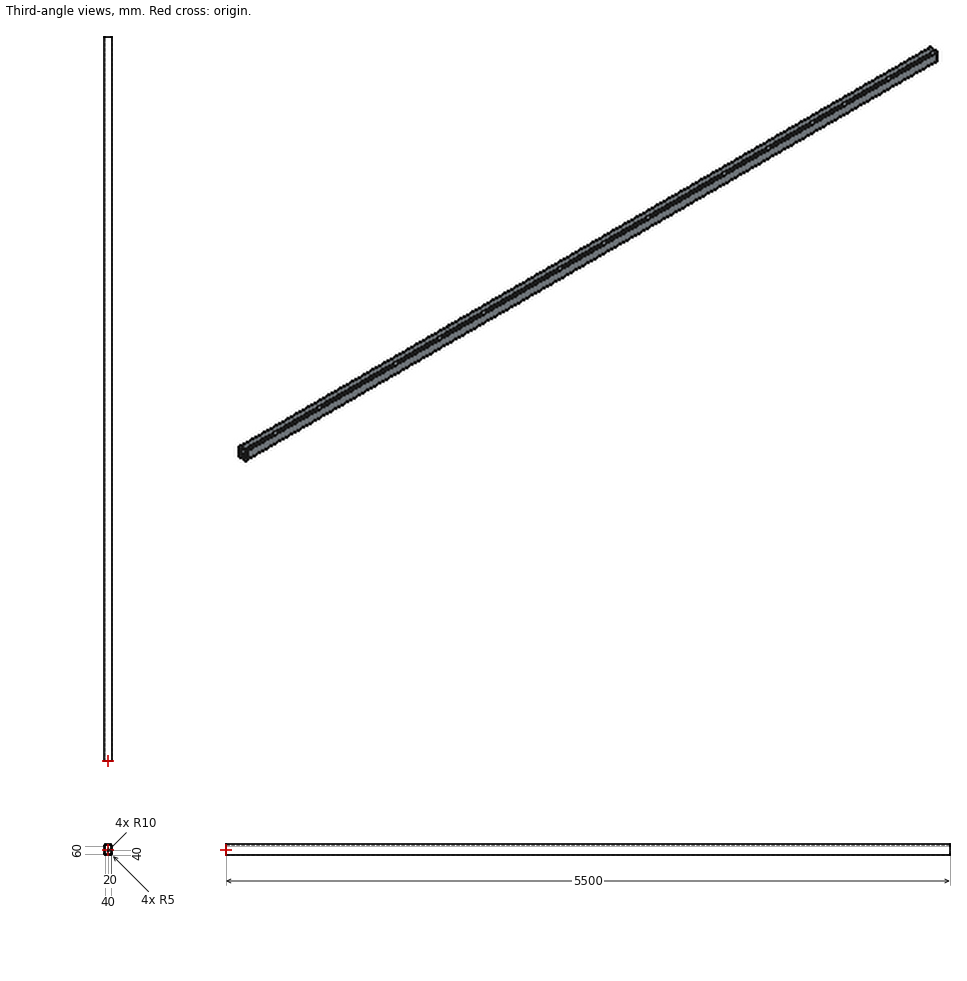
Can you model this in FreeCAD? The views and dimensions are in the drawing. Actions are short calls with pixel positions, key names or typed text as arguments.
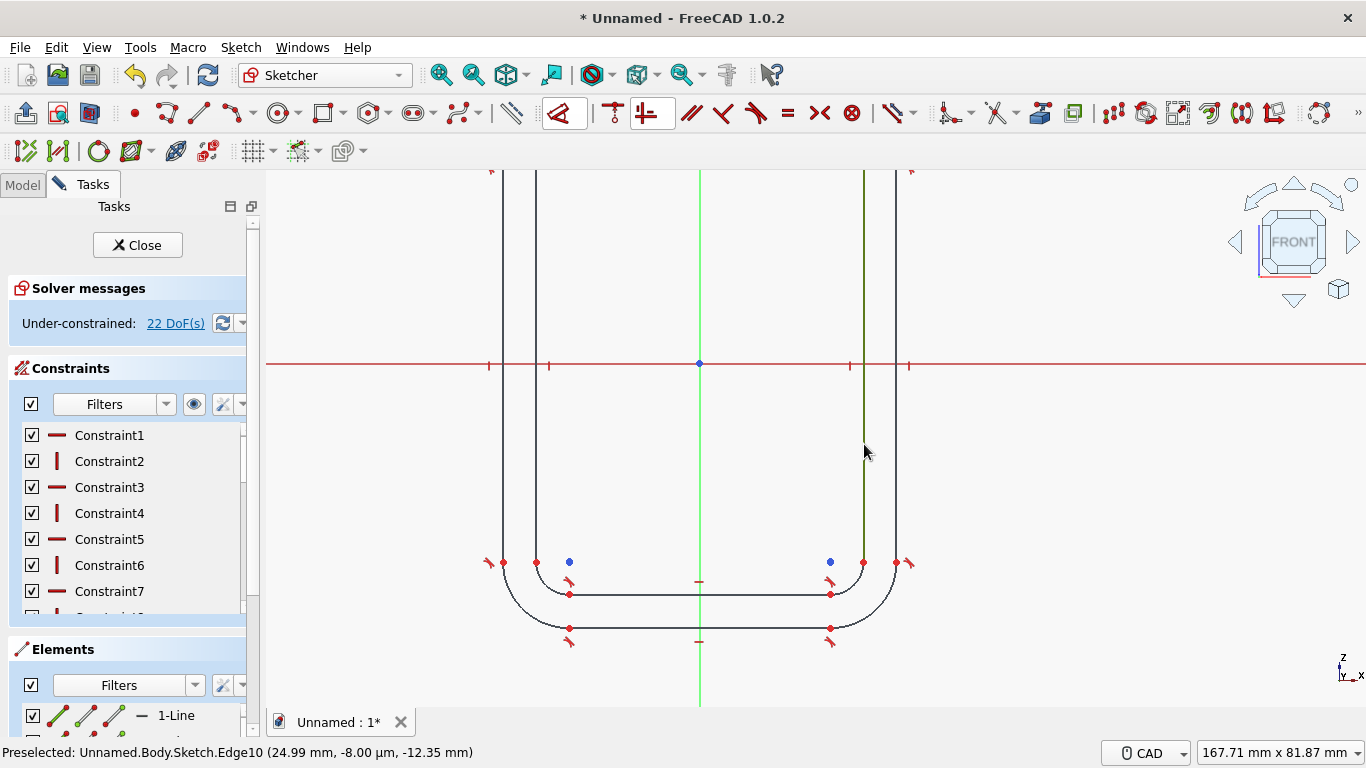
click(845, 591)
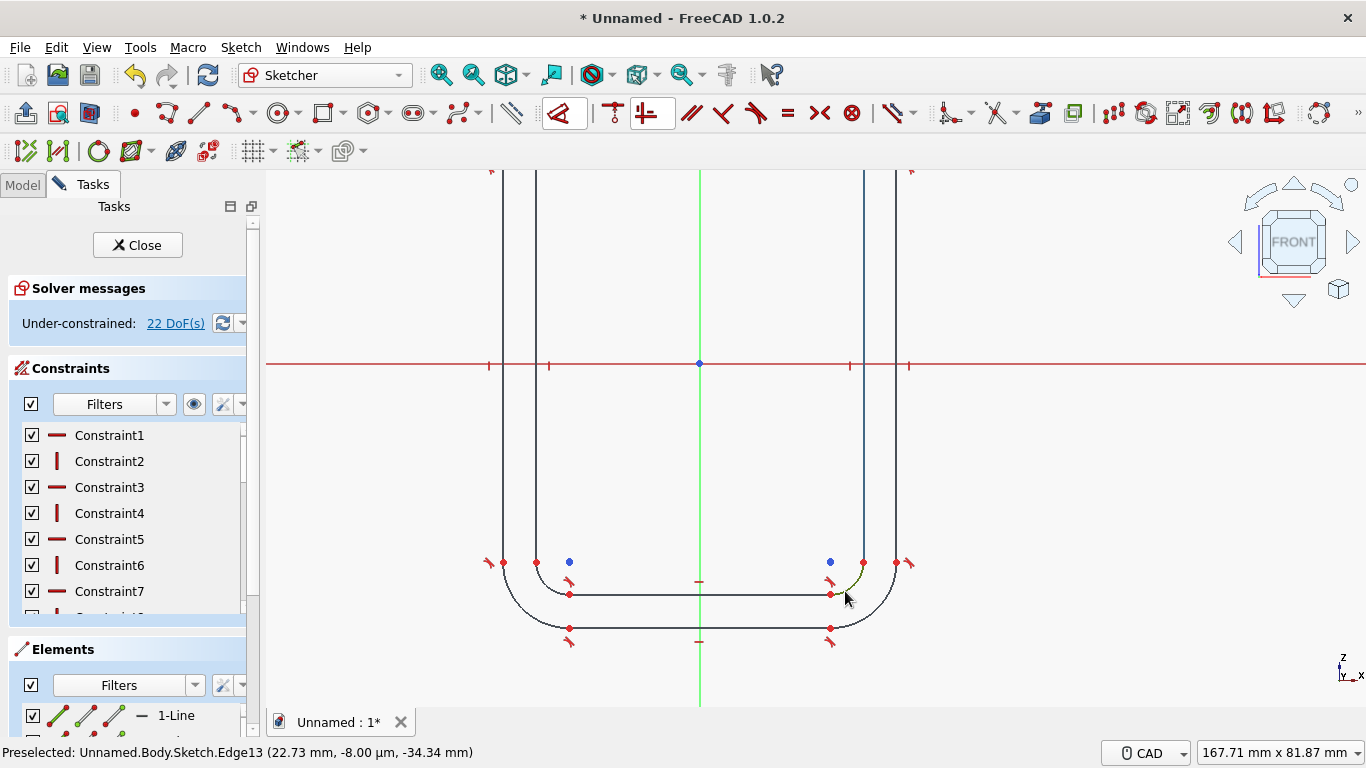
click(756, 114)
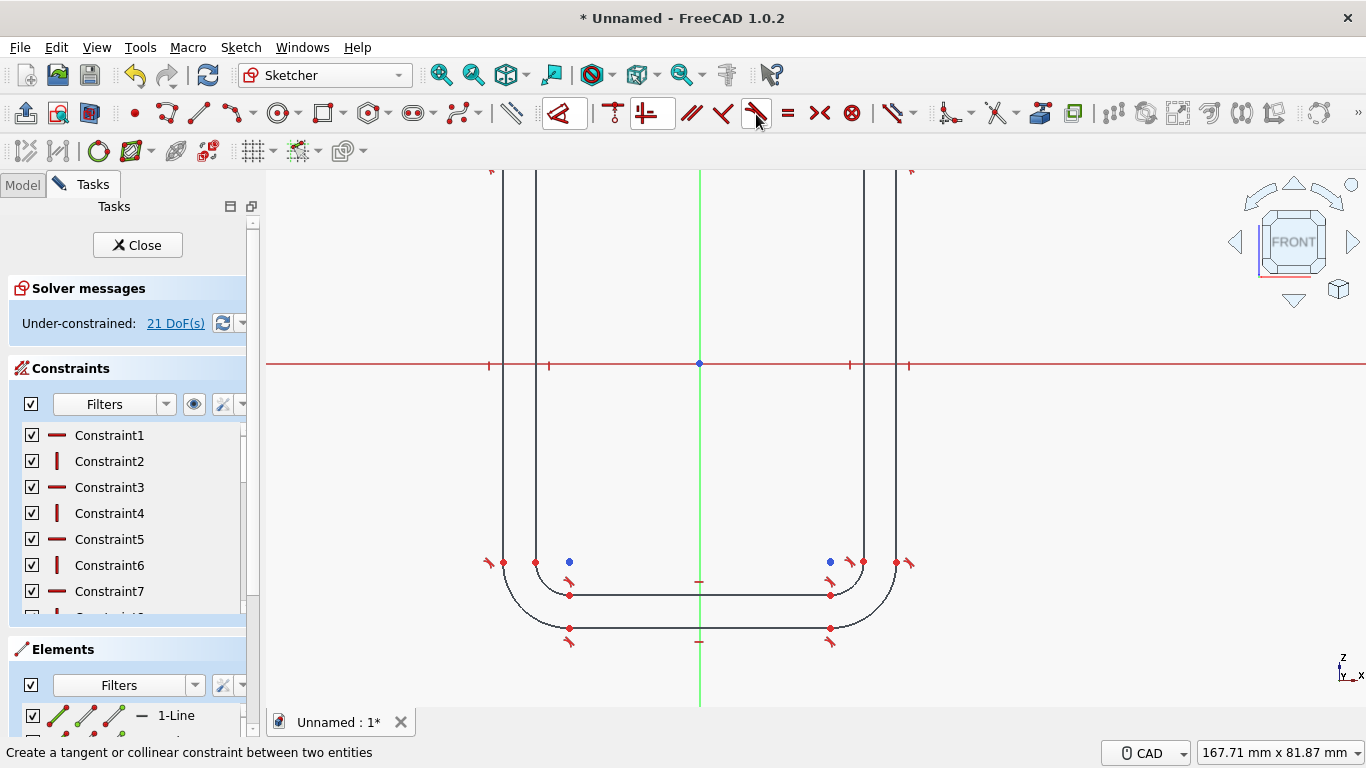
click(864, 444)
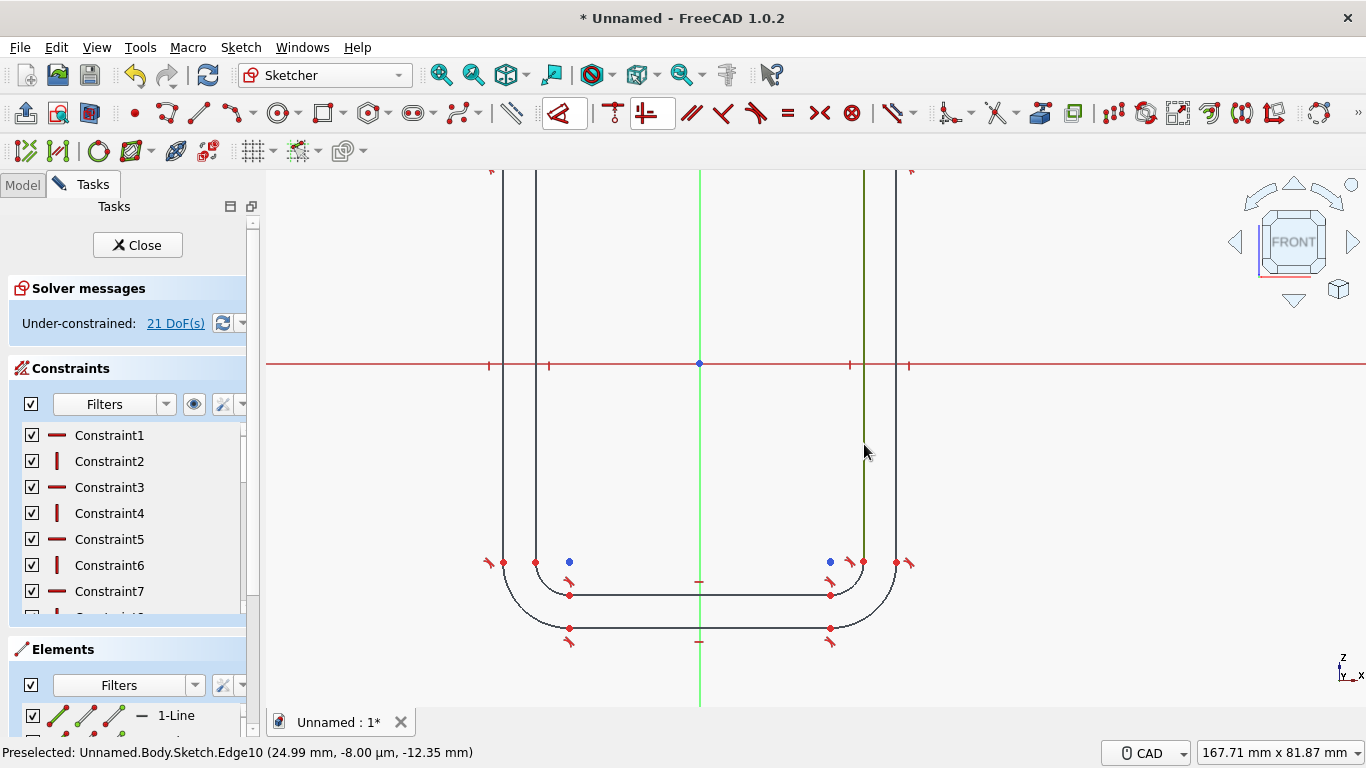
scroll(844, 590, down, 2)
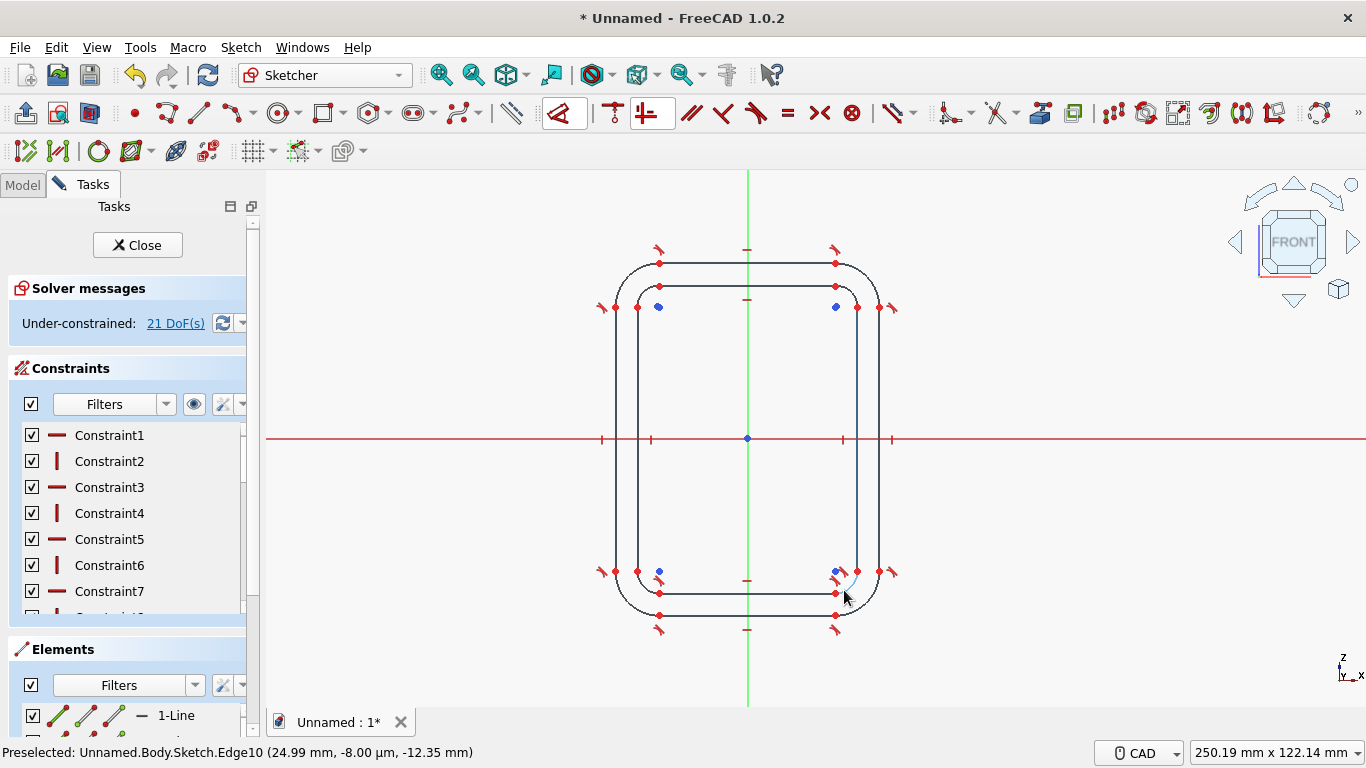
scroll(855, 297, up, 2)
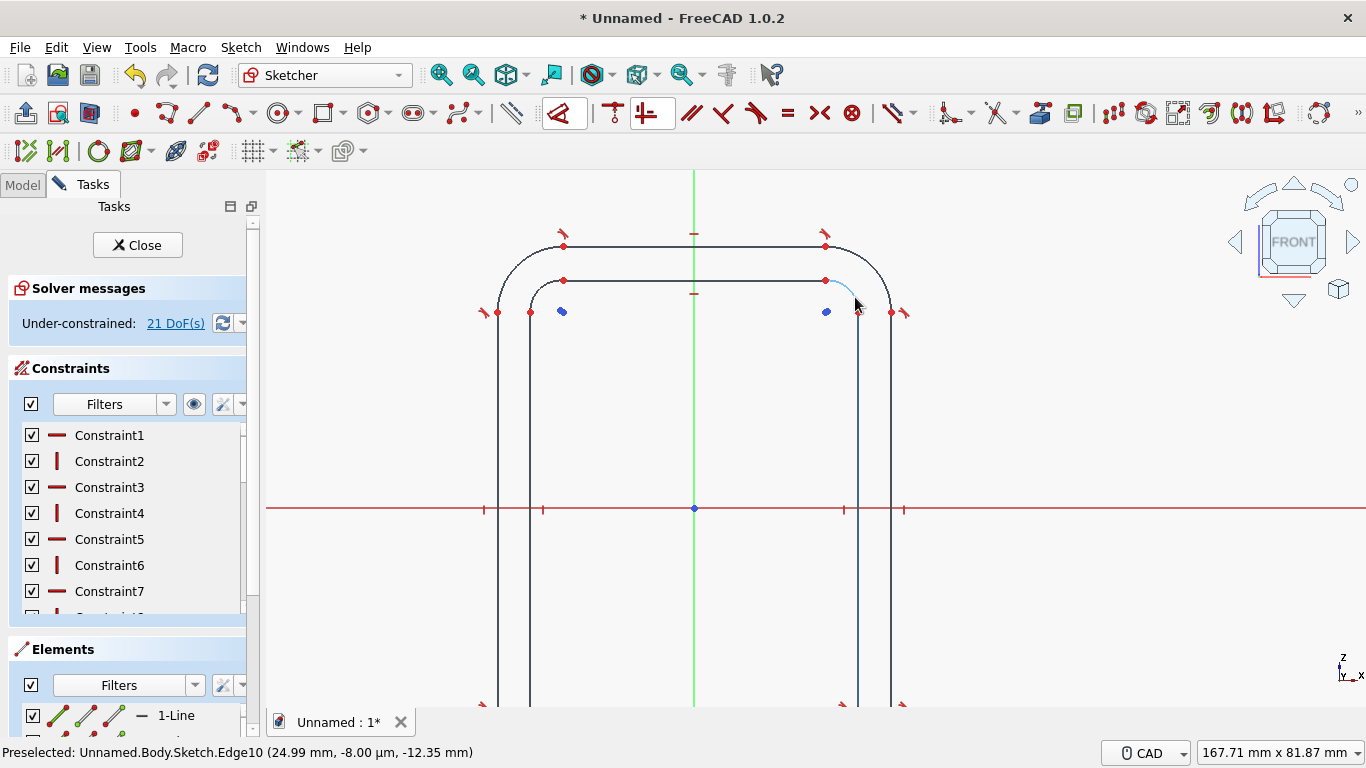
click(855, 297)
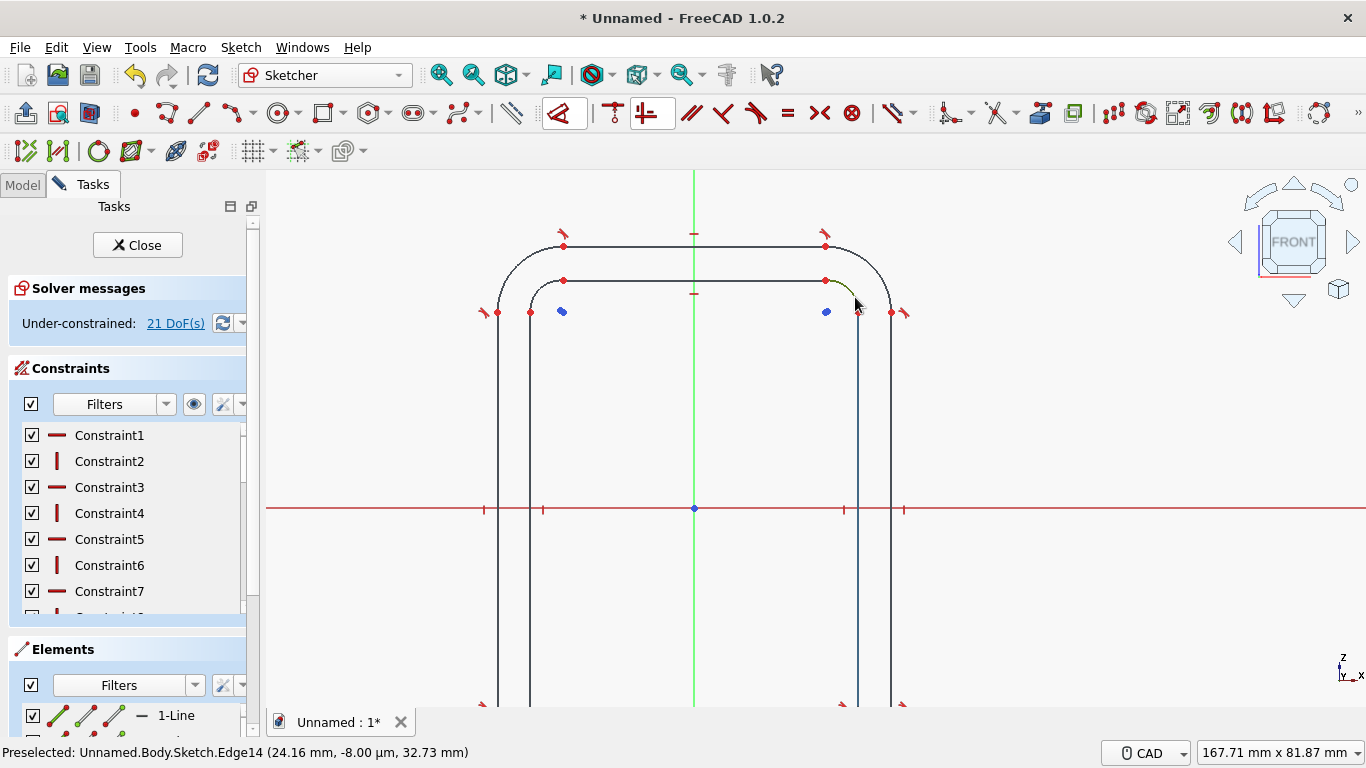
click(756, 114)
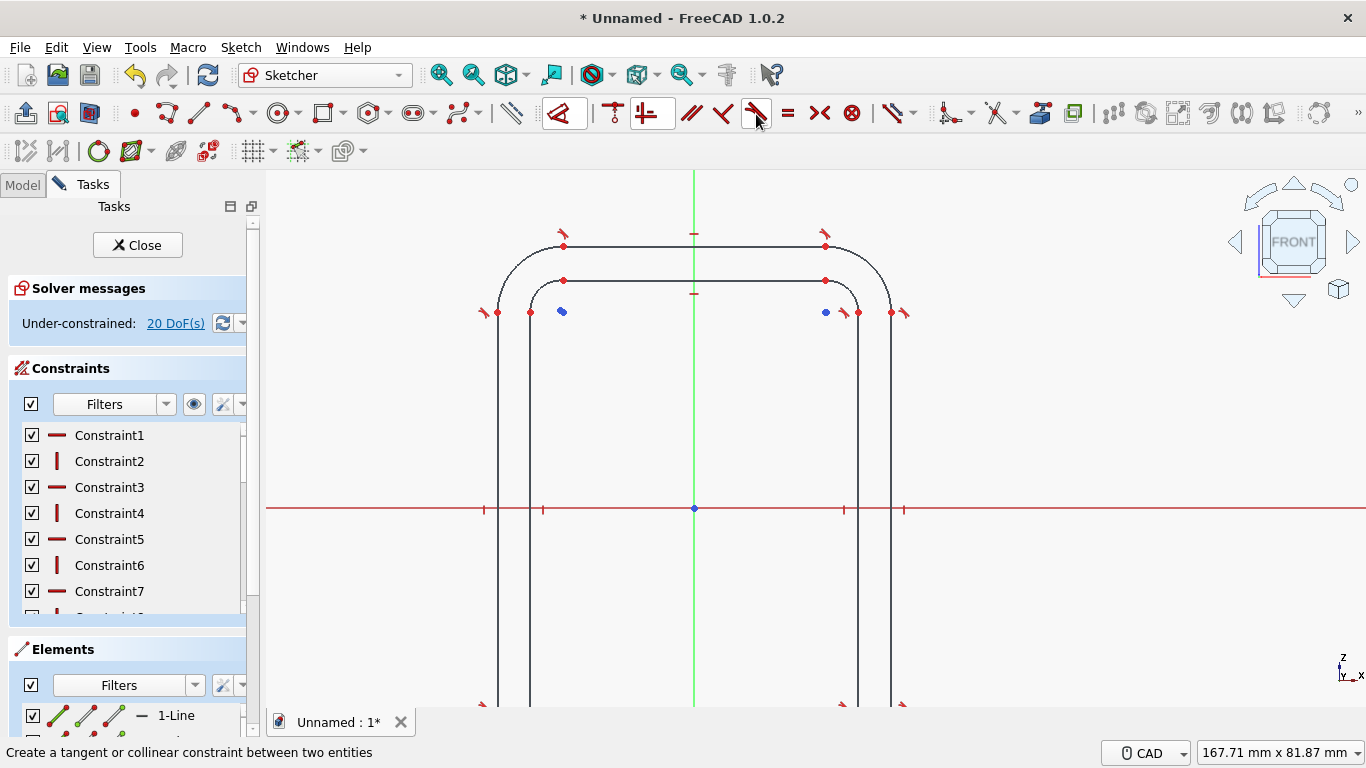
click(747, 281)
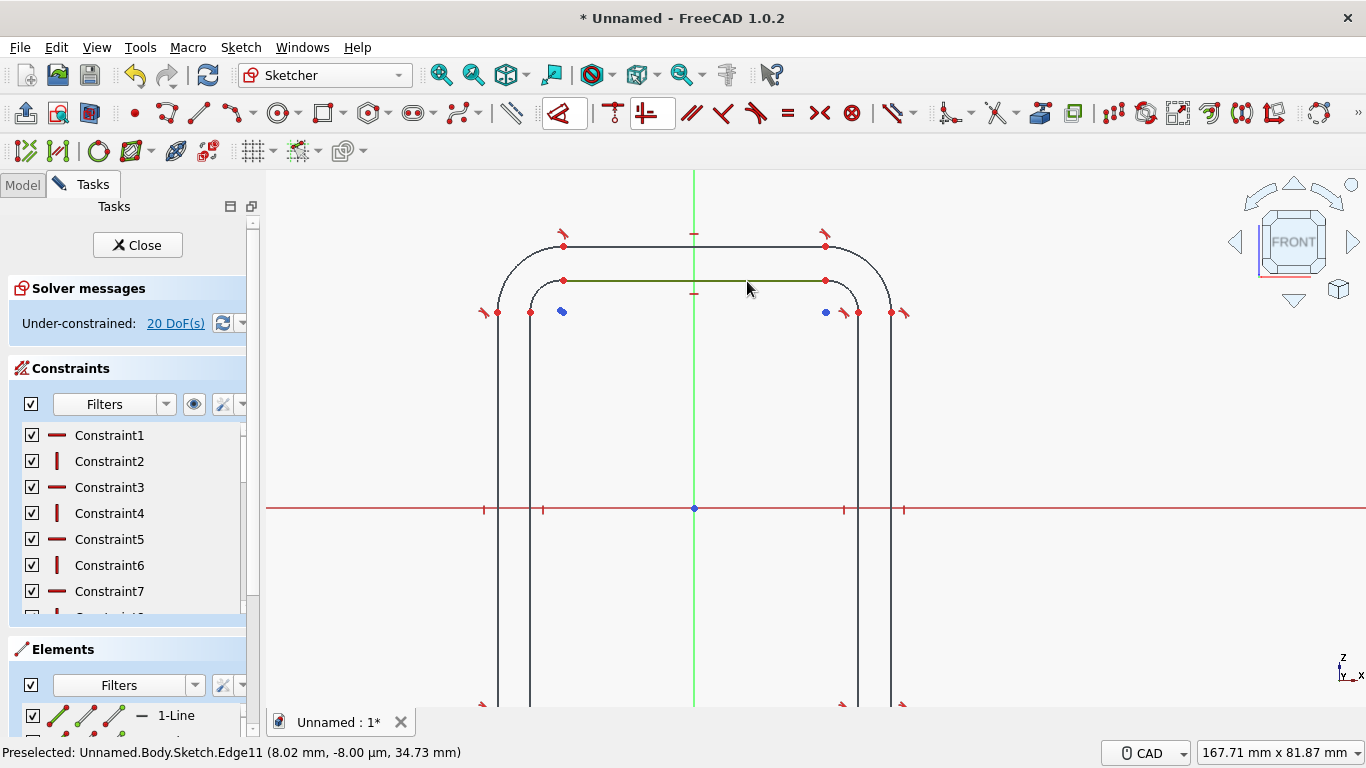
click(855, 297)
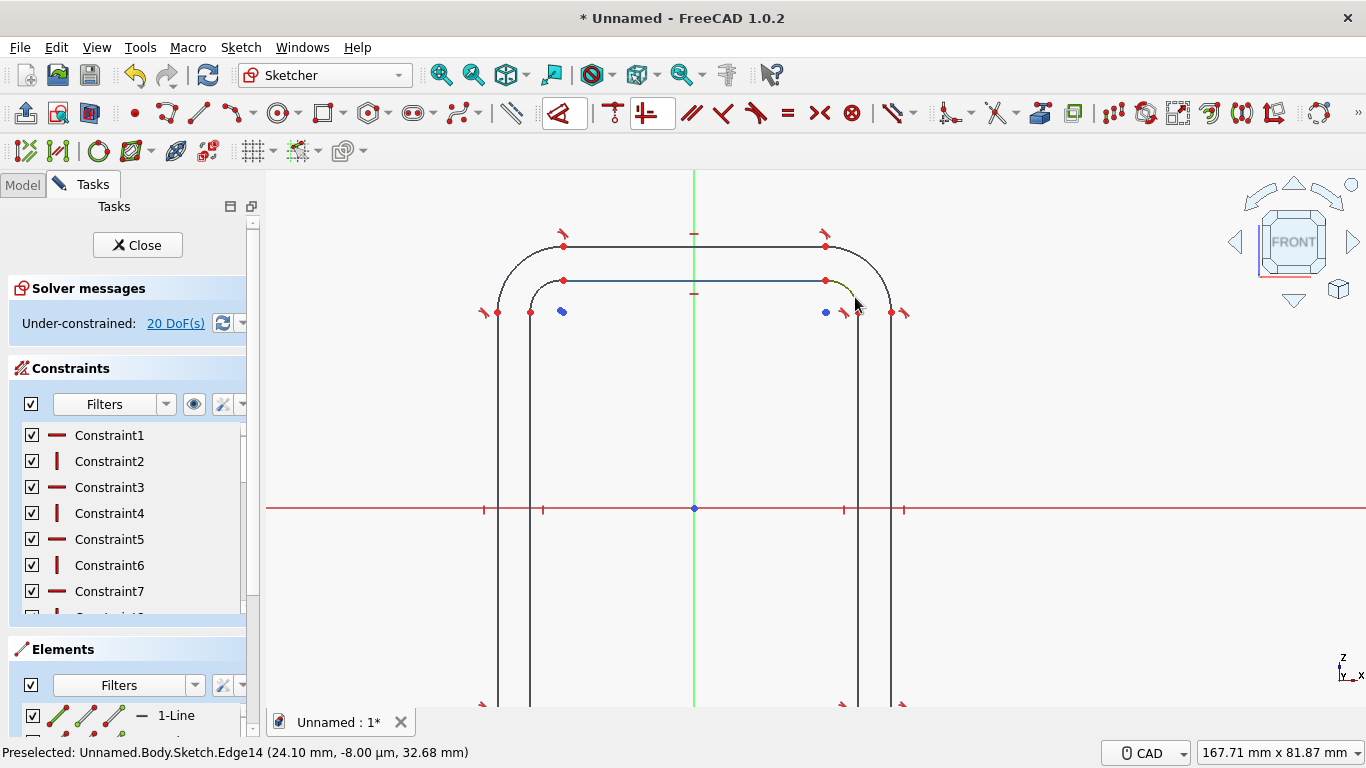
click(756, 114)